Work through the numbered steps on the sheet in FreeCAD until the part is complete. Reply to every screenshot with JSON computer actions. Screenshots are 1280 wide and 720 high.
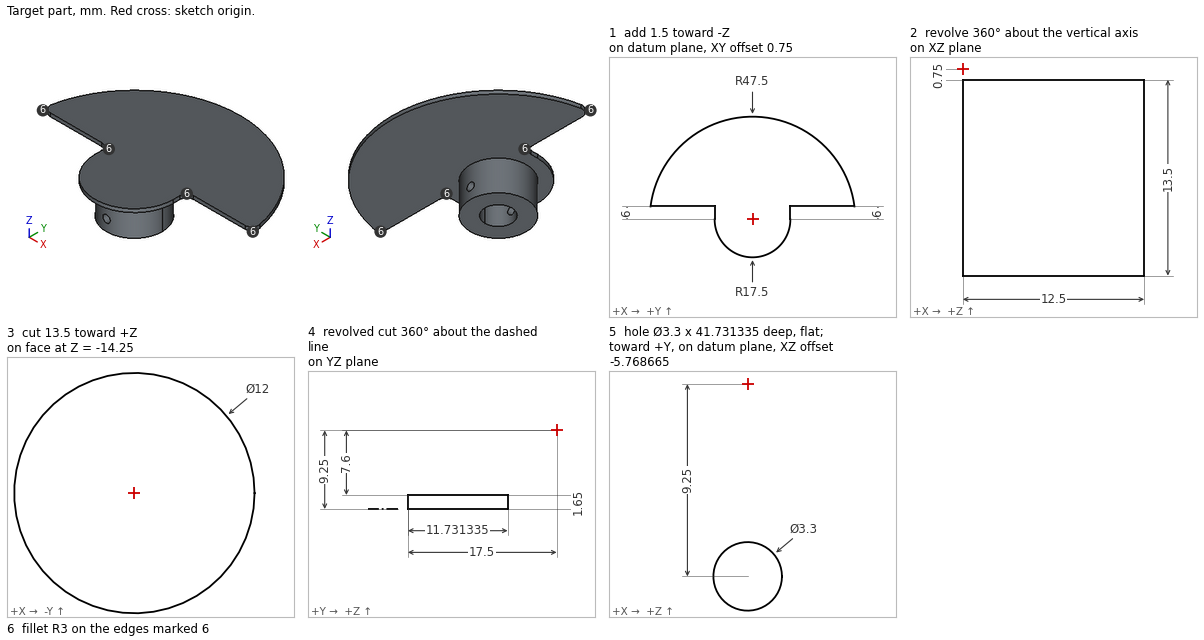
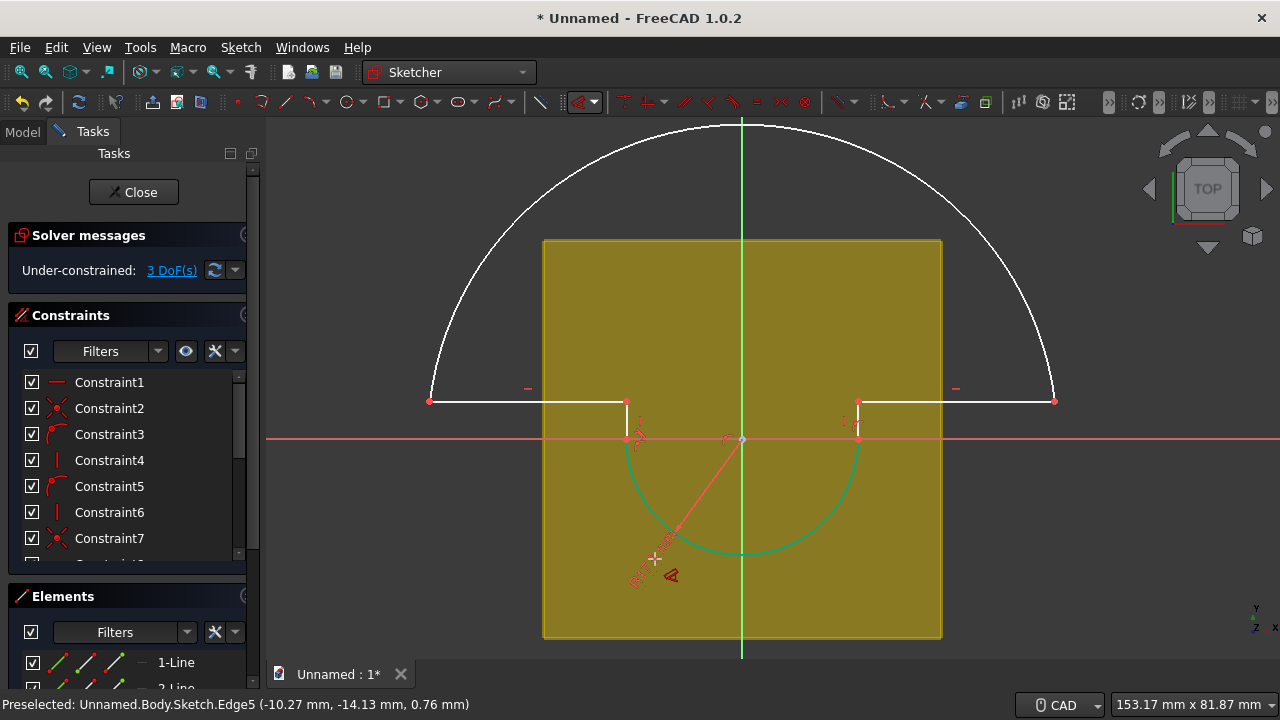
{"action": "left_click", "coordinate": [915, 176]}
{"action": "left_click", "coordinate": [933, 149]}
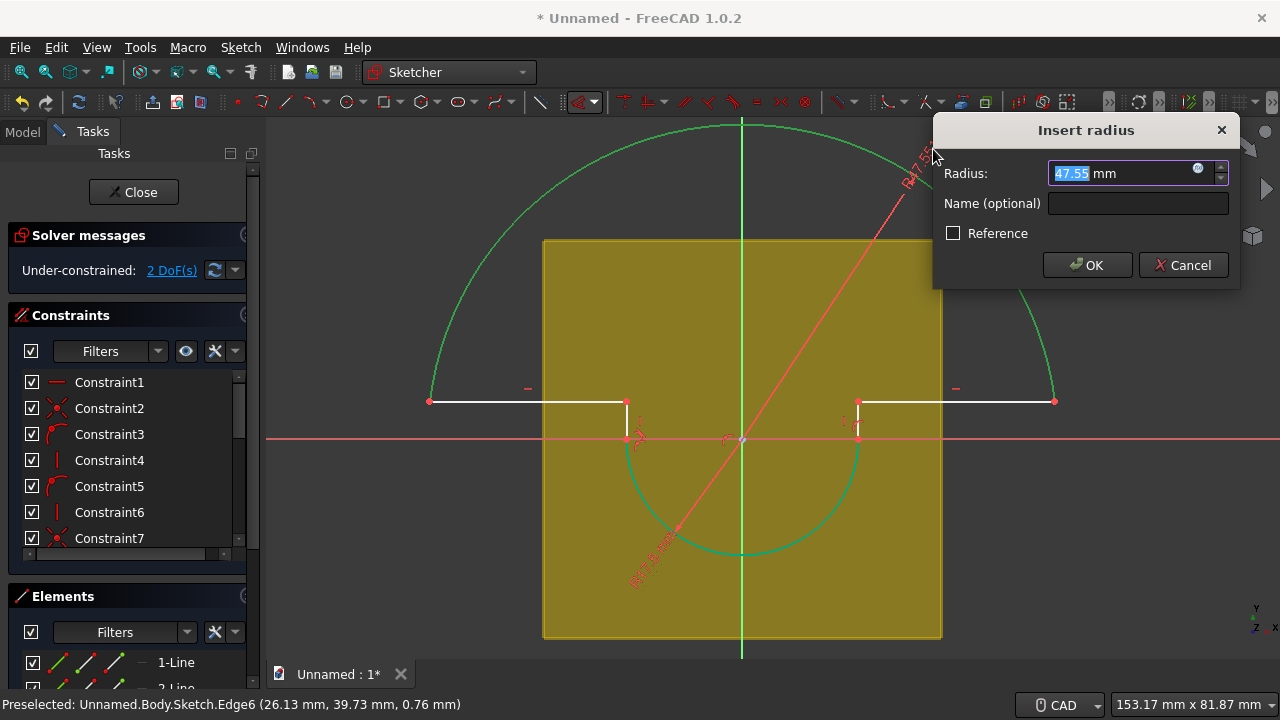
{"action": "type", "text": "47.5"}
{"action": "key", "text": "Return"}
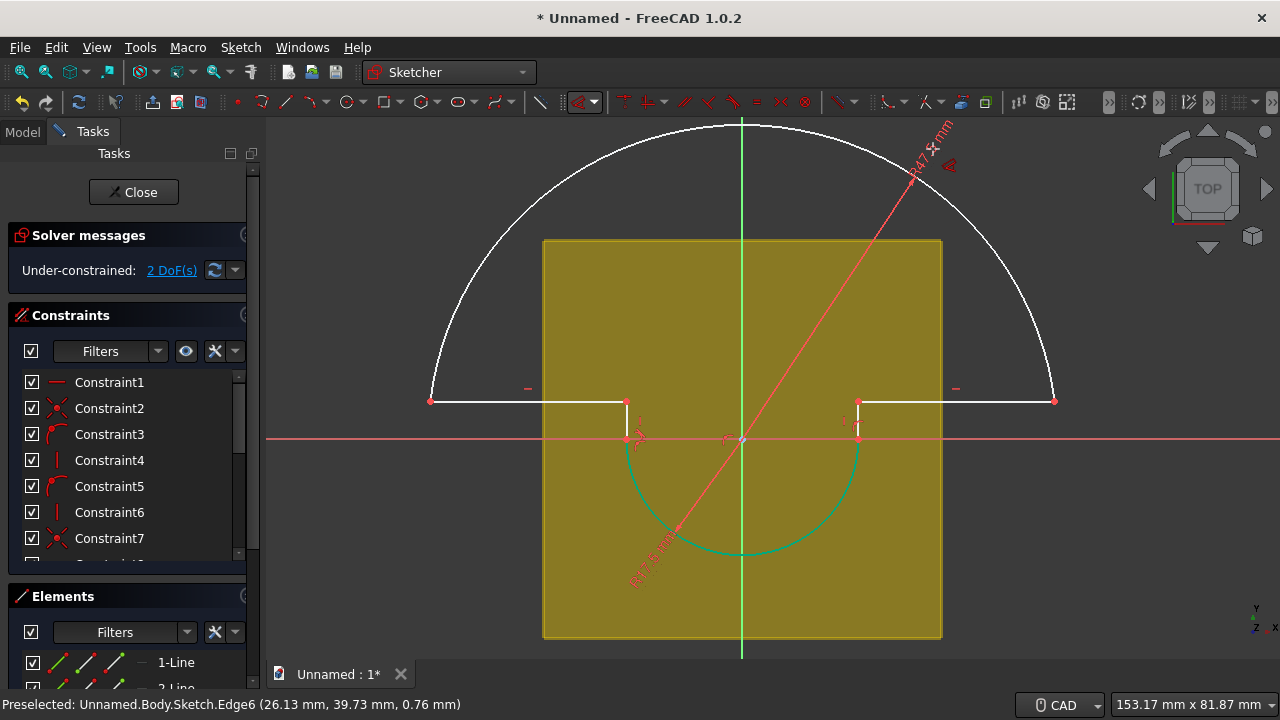
{"action": "scroll", "coordinate": [627, 413], "scroll_direction": "up", "scroll_amount": 2}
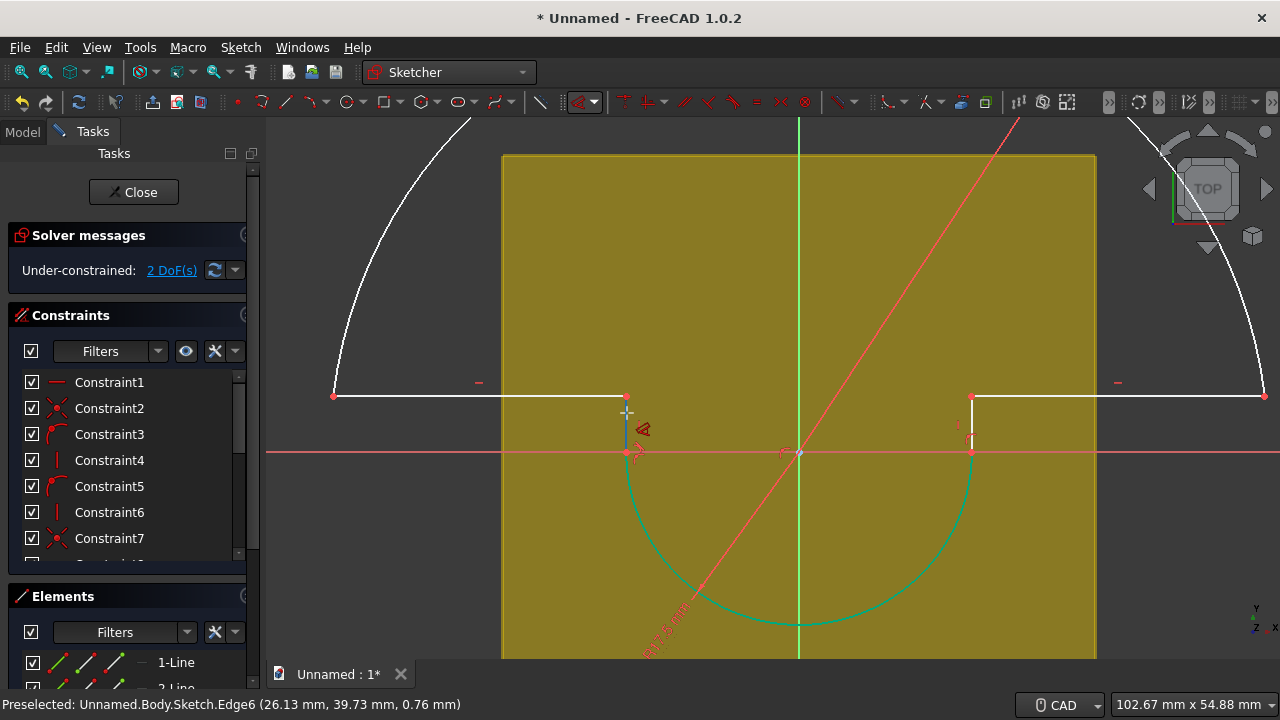
{"action": "left_click", "coordinate": [626, 413]}
{"action": "left_click", "coordinate": [592, 424]}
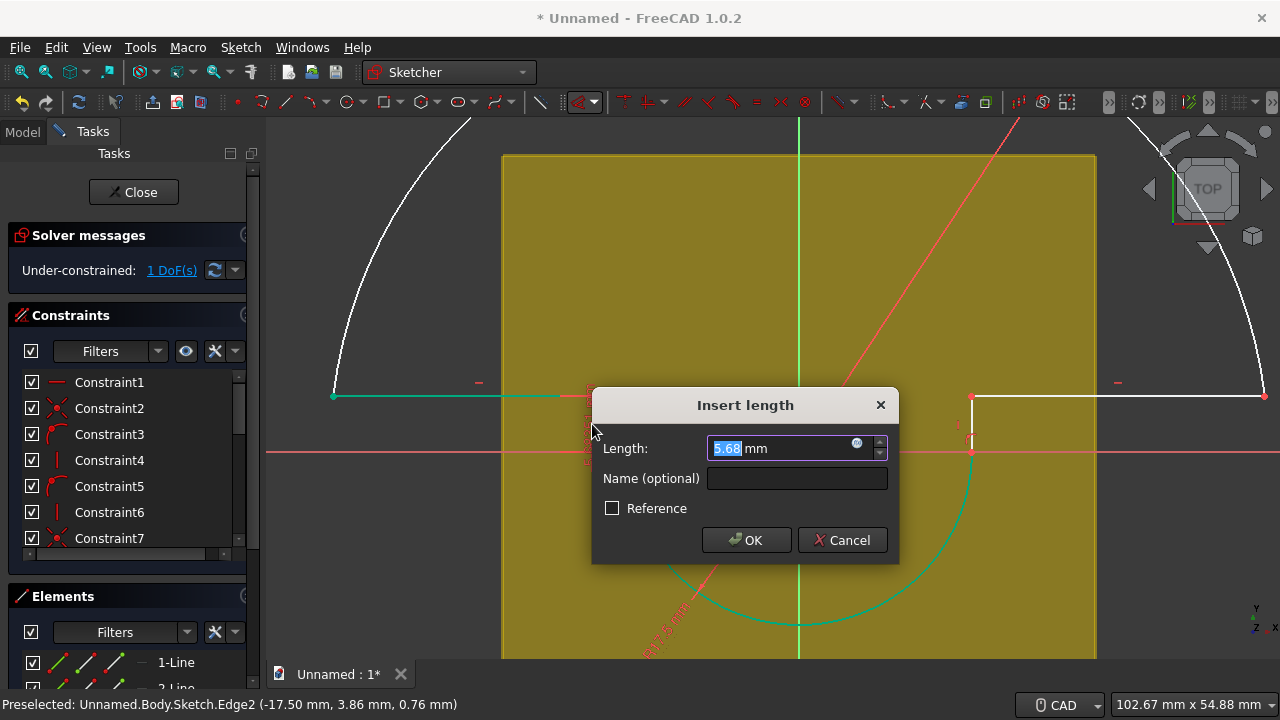
{"action": "type", "text": "6"}
{"action": "key", "text": "Return"}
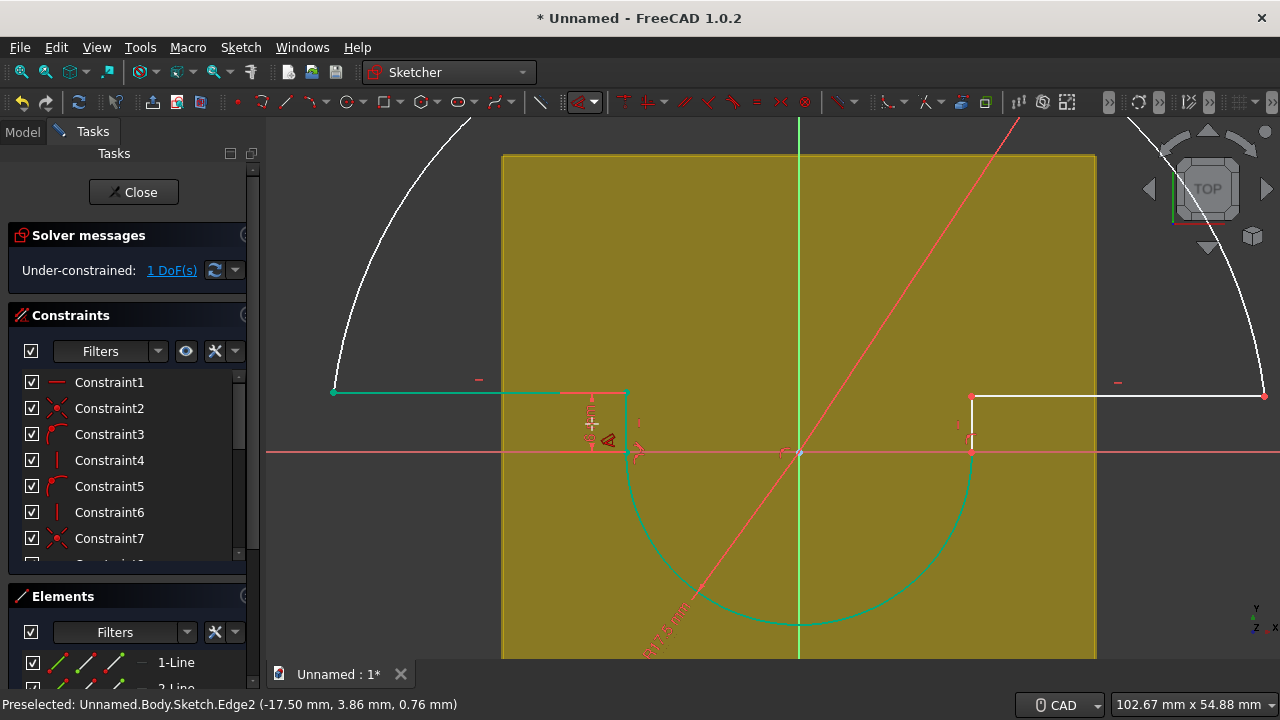
{"action": "left_click", "coordinate": [972, 435]}
{"action": "left_click", "coordinate": [1006, 424]}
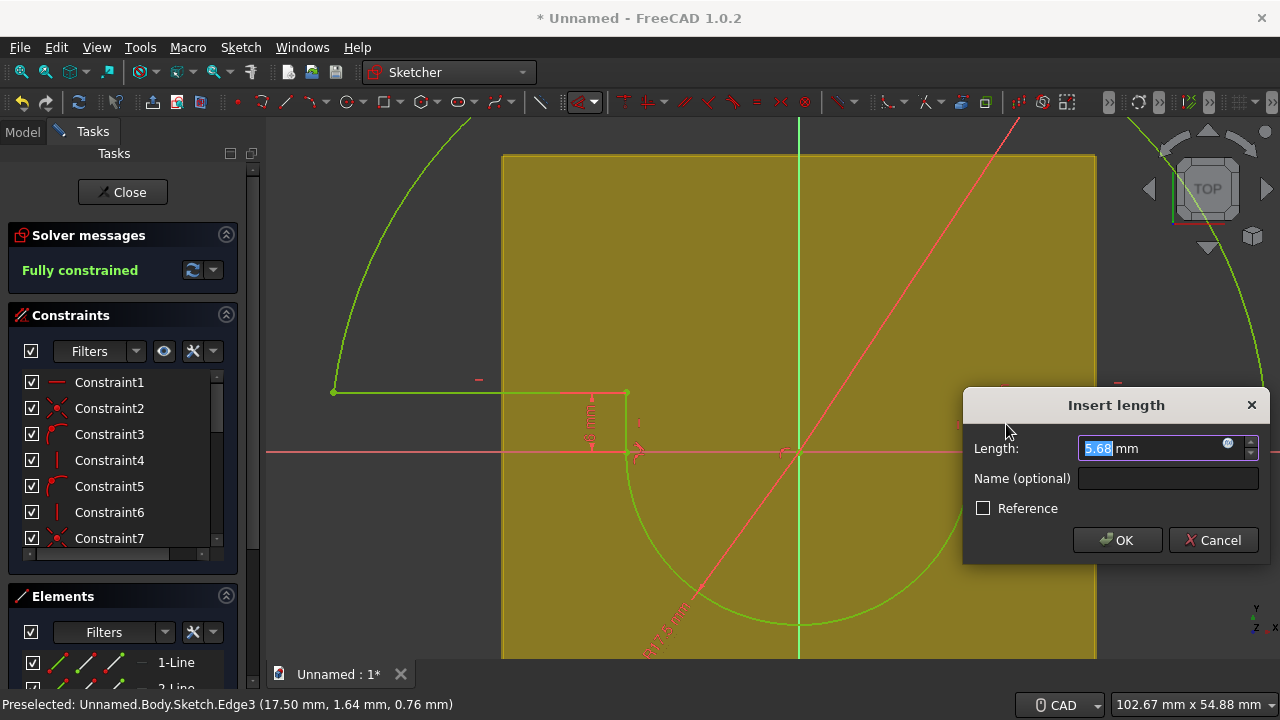
{"action": "type", "text": "6"}
{"action": "key", "text": "Return"}
{"action": "key", "text": "Escape"}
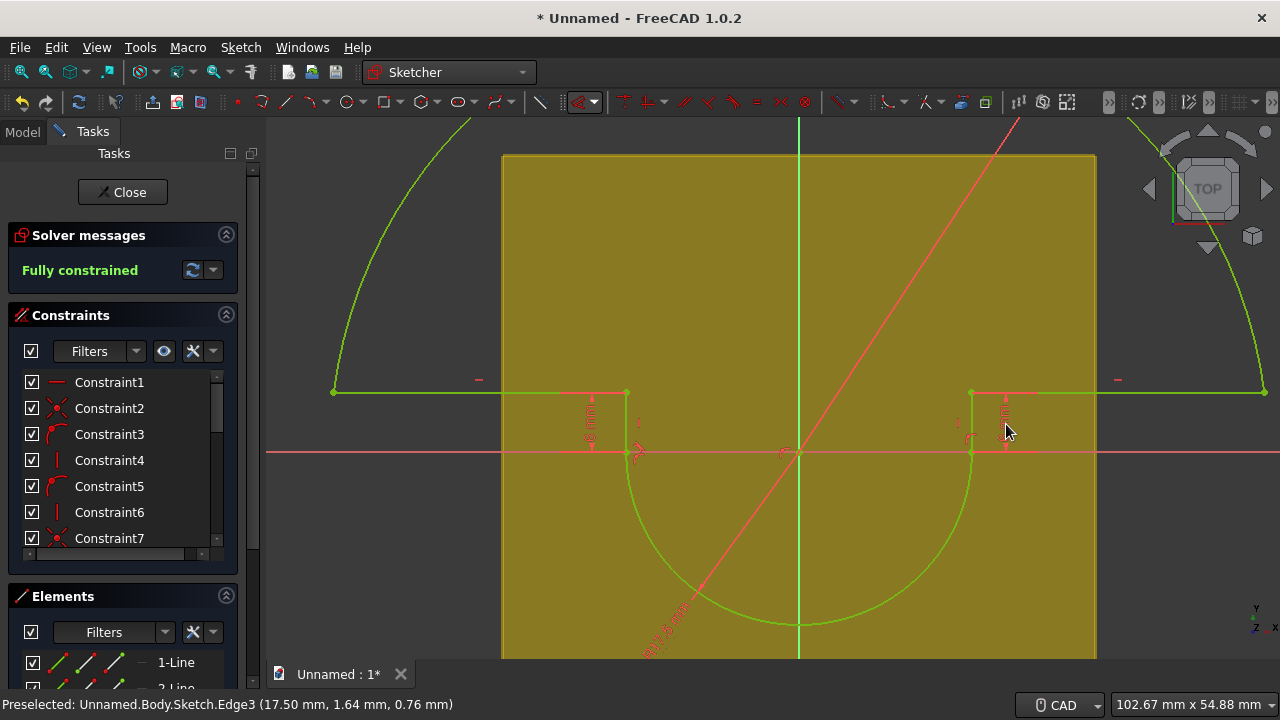
{"action": "left_click", "coordinate": [123, 192]}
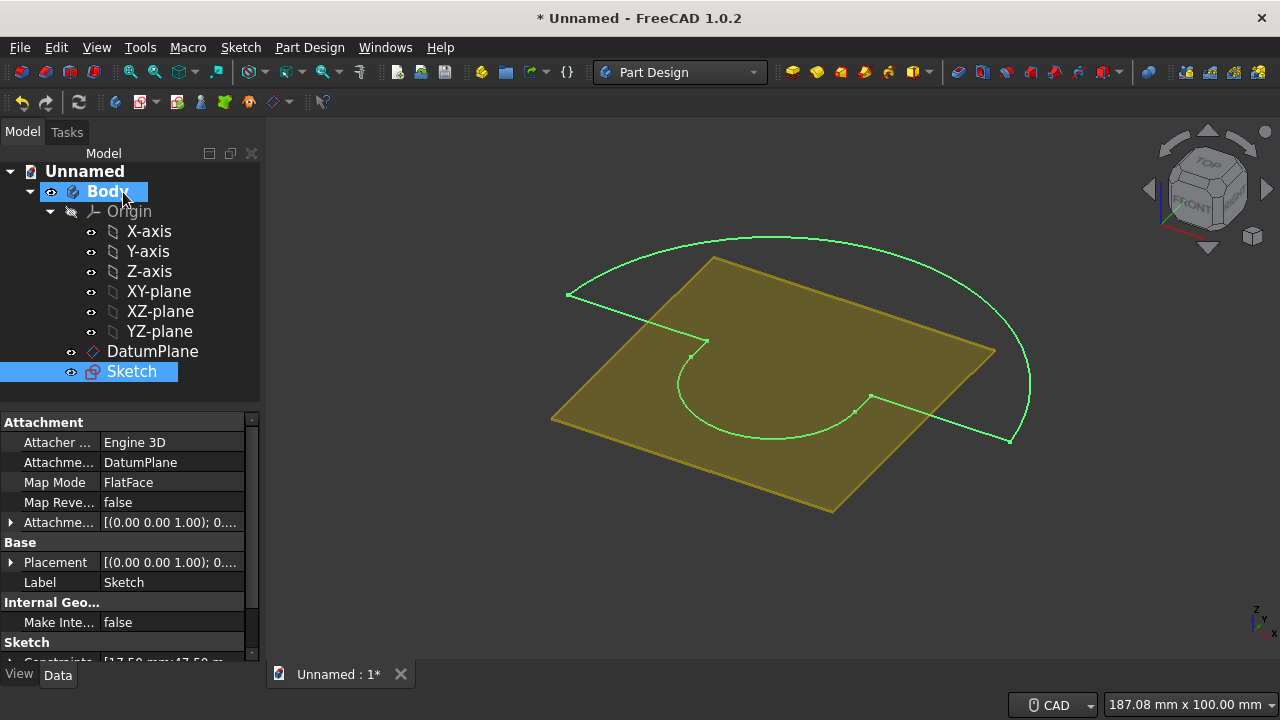
{"action": "left_click", "coordinate": [794, 72]}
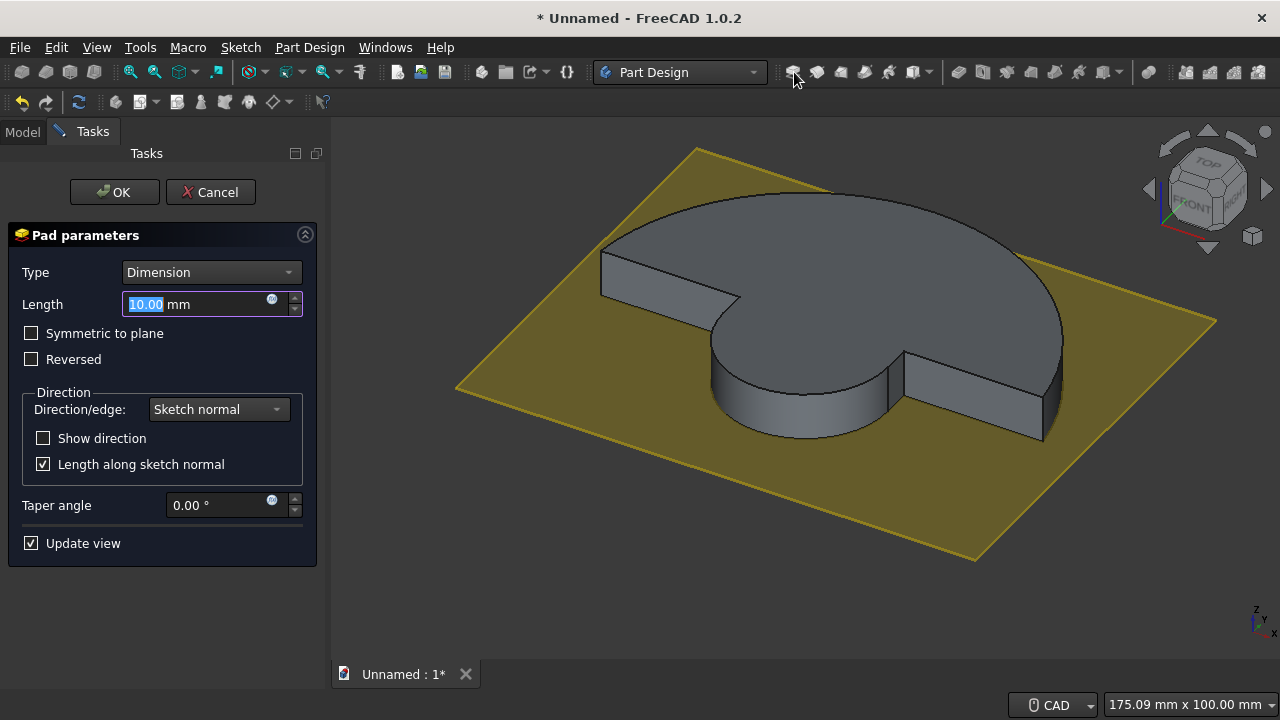
{"action": "type", "text": "1.5"}
{"action": "key", "text": "Tab"}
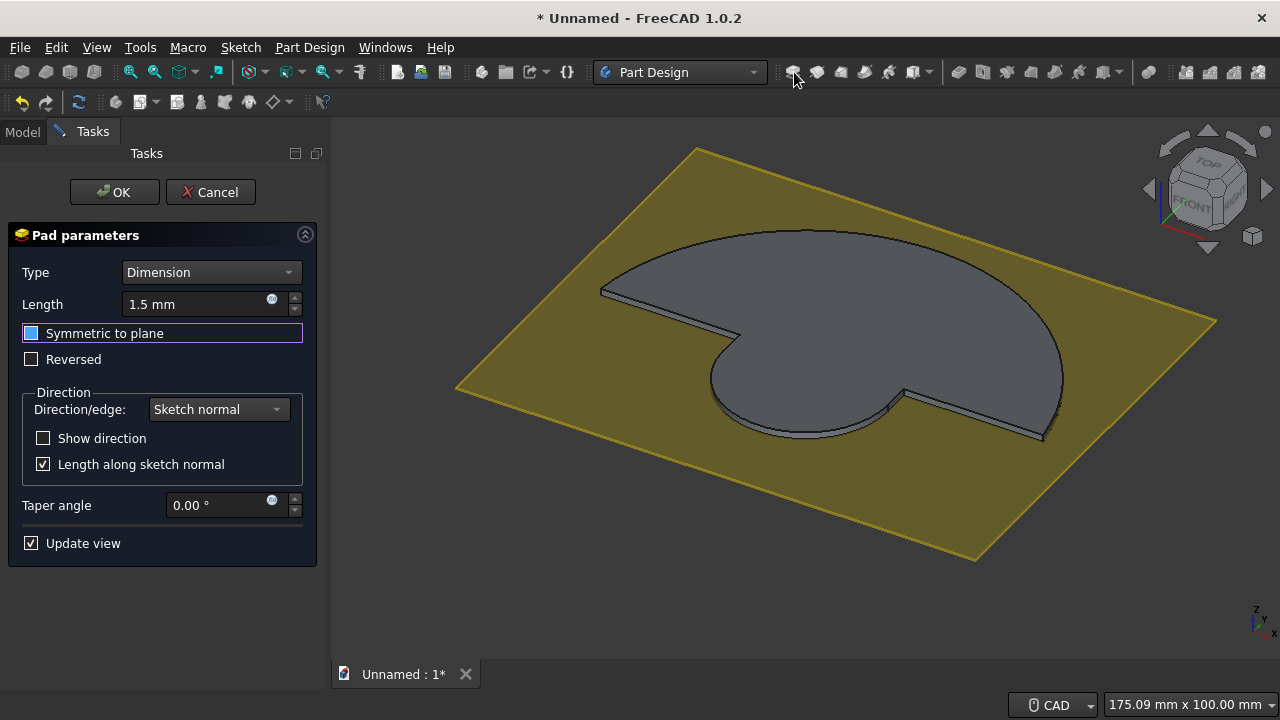
{"action": "left_click", "coordinate": [30, 359]}